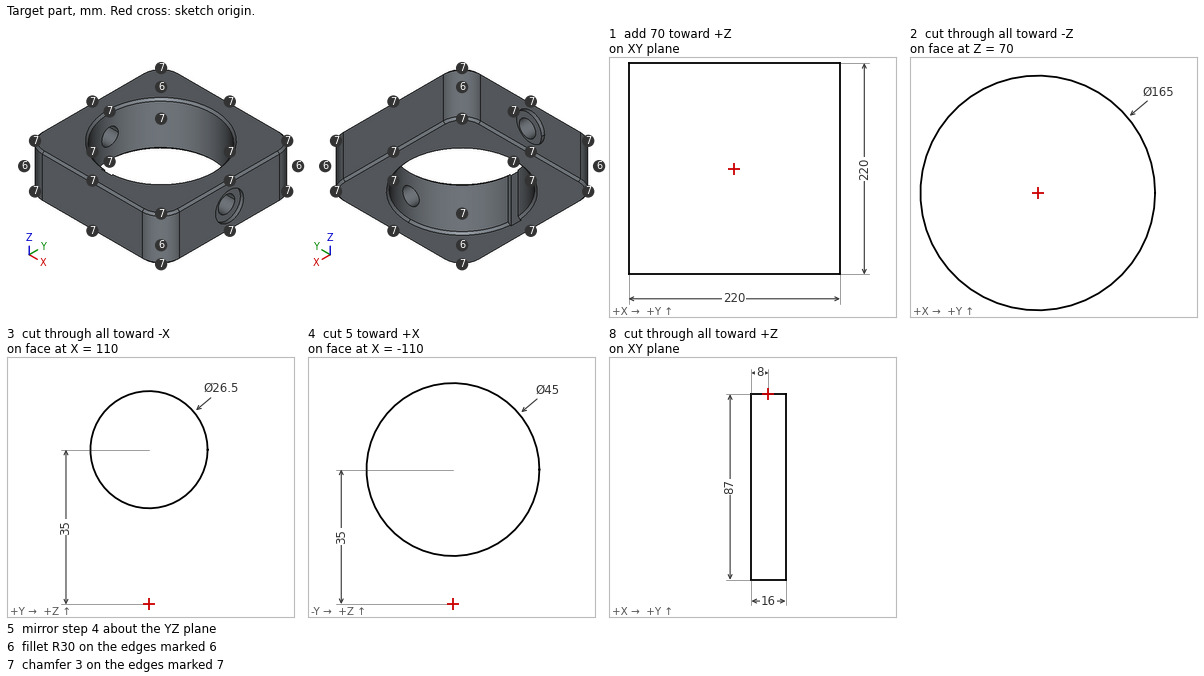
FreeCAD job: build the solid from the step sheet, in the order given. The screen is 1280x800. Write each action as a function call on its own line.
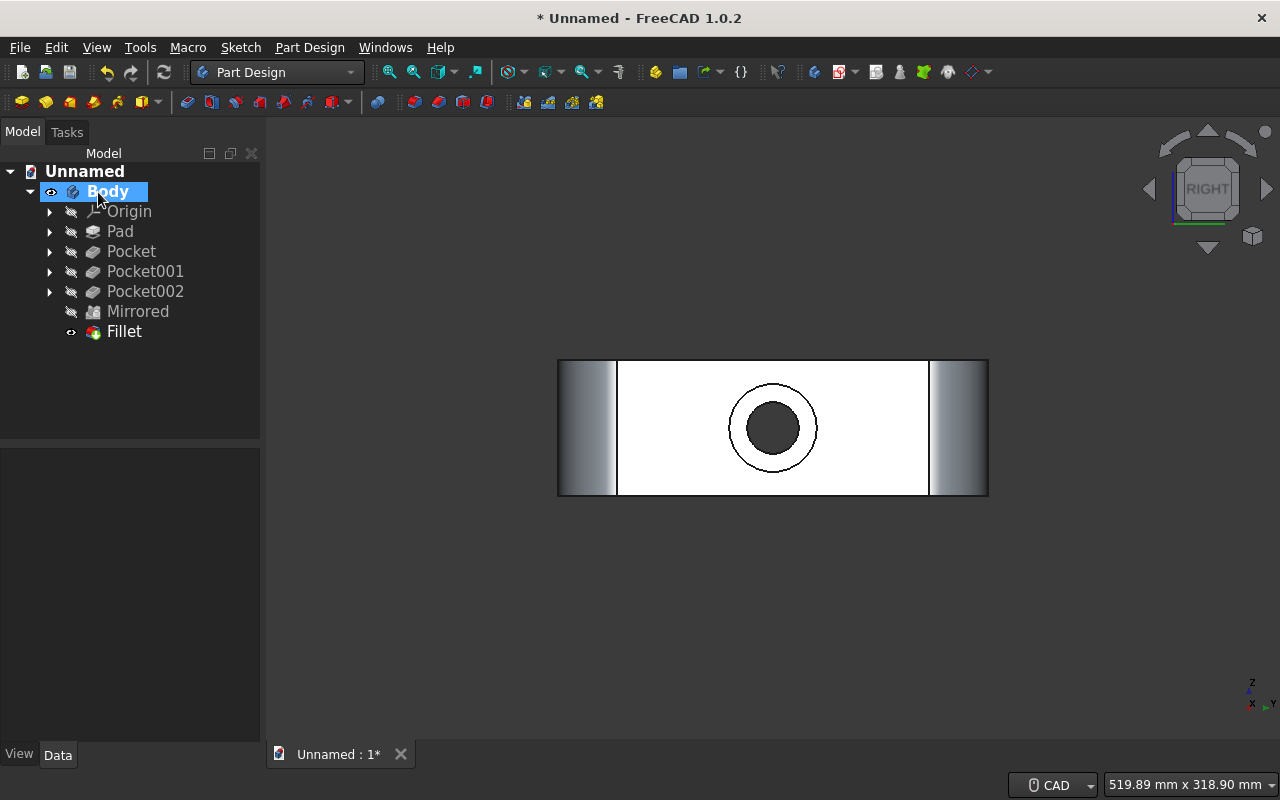
key(v)
key(f)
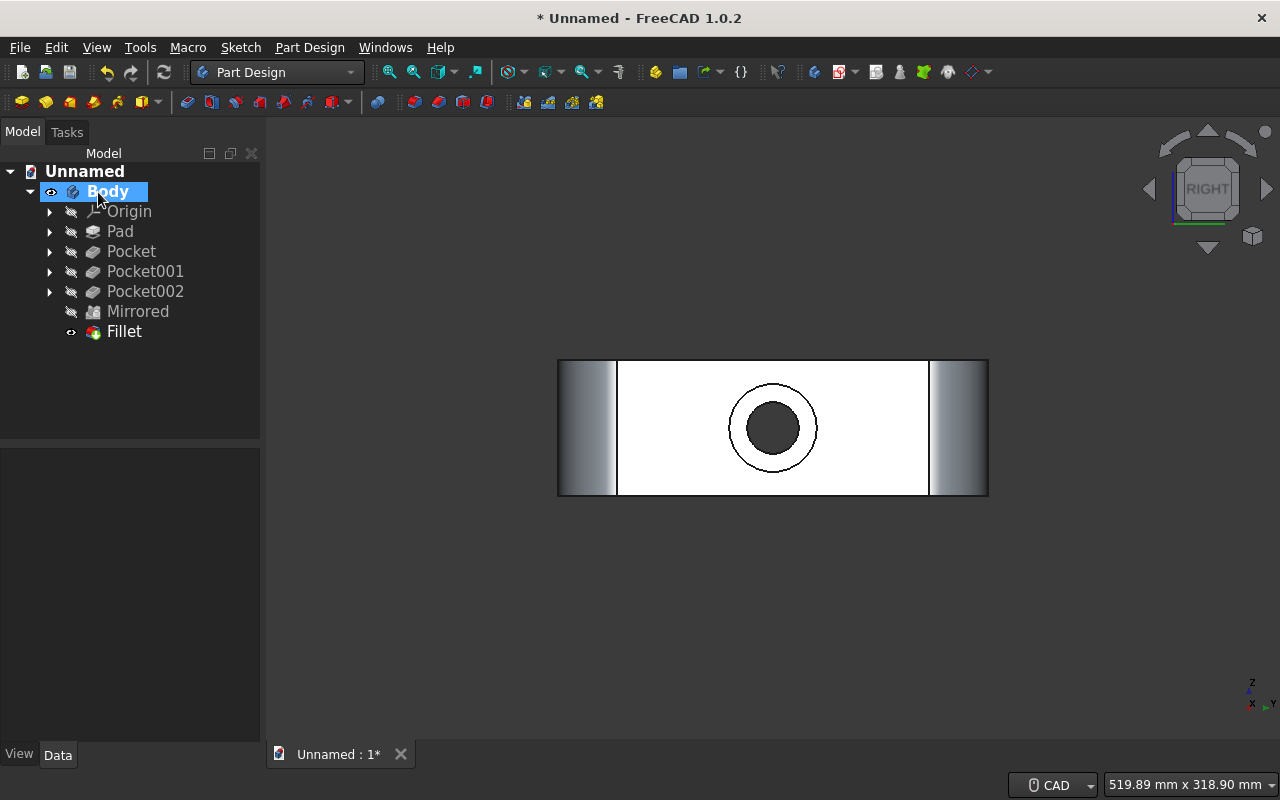
key(0)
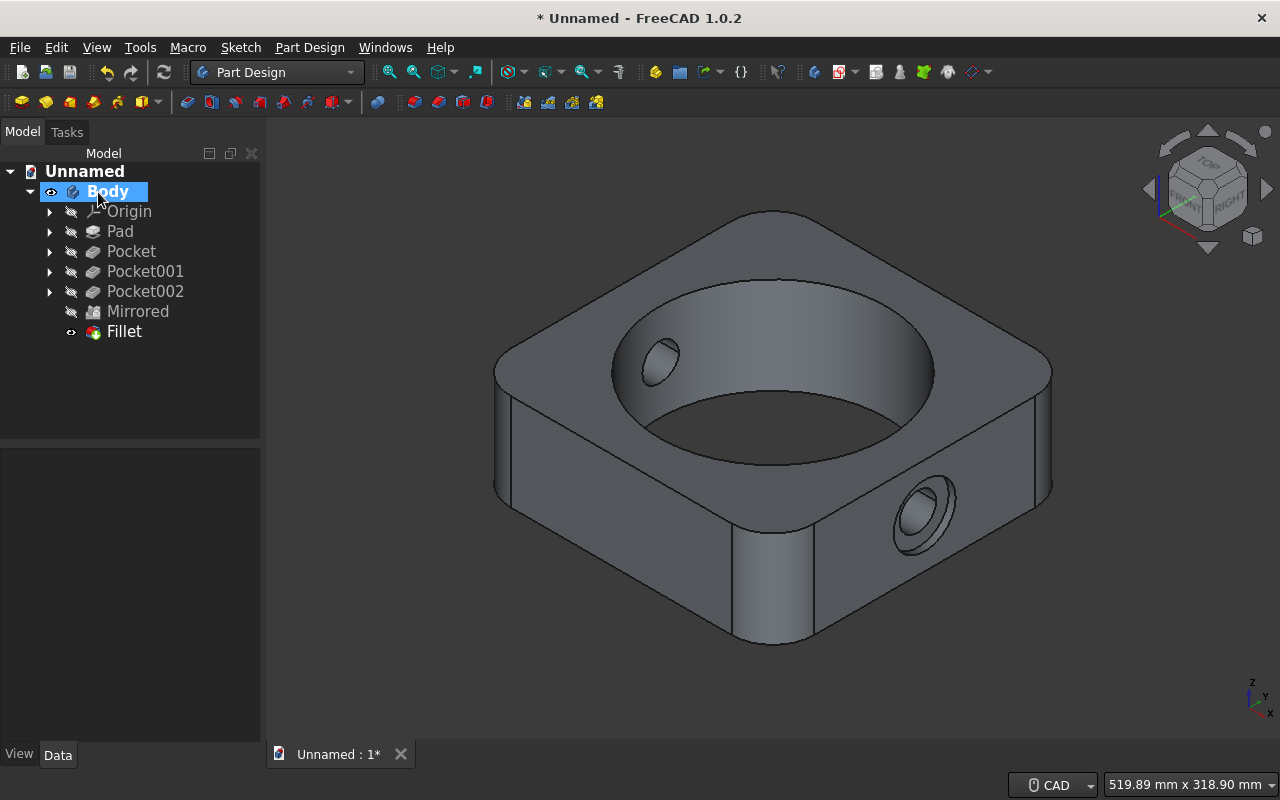
click(990, 396)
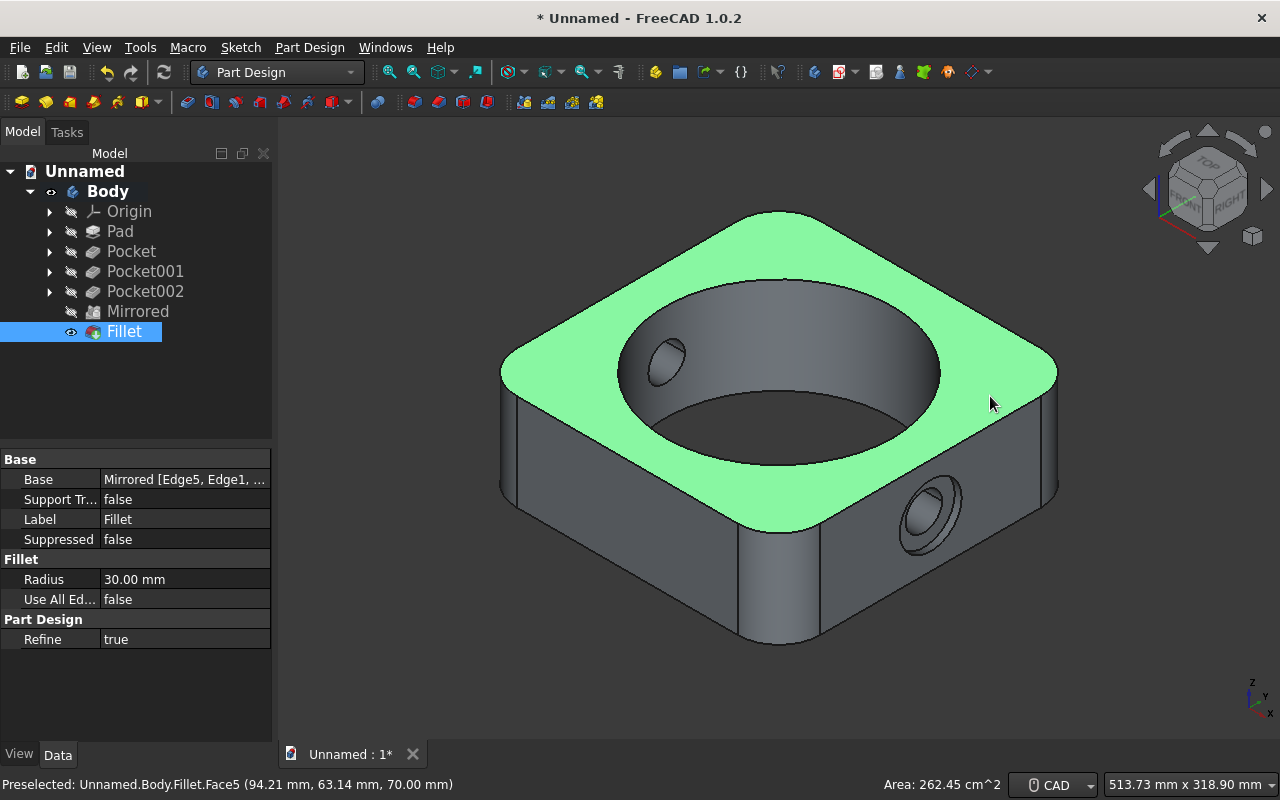
key(2)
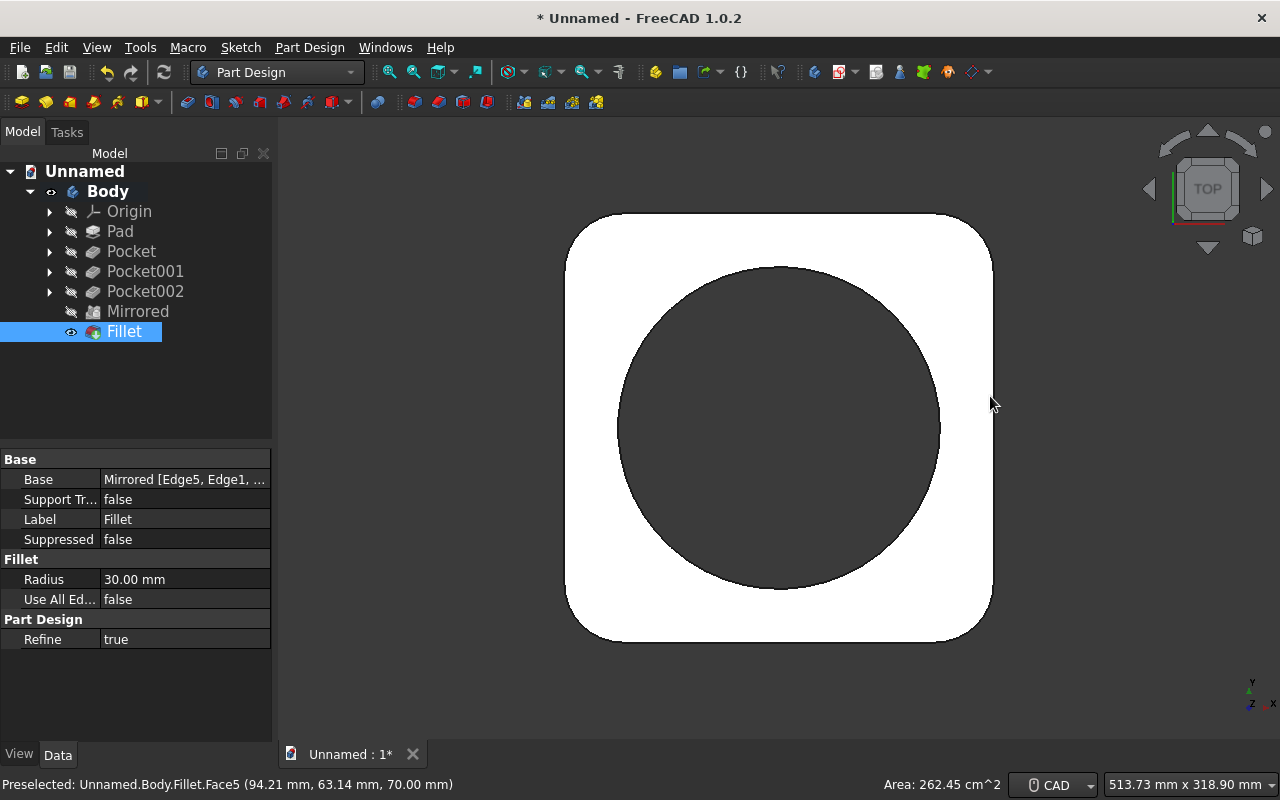
key(1)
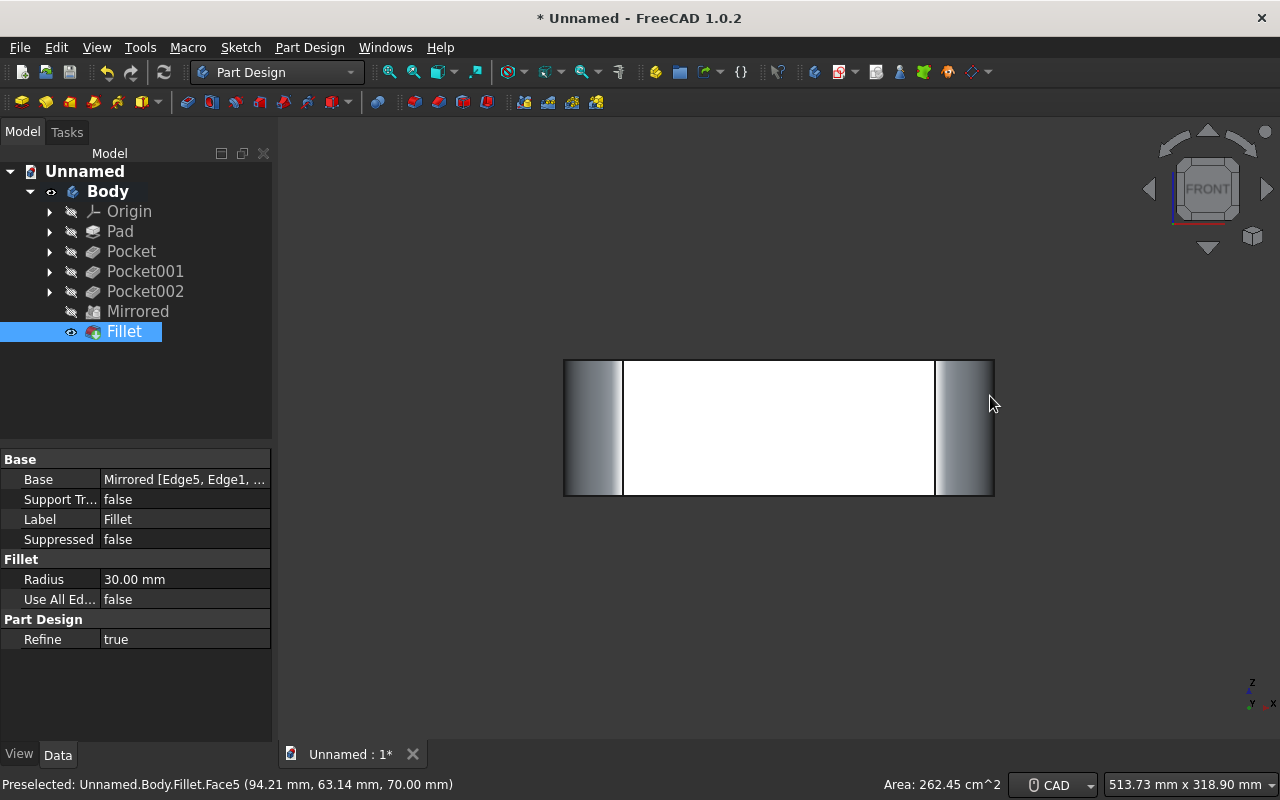
click(390, 72)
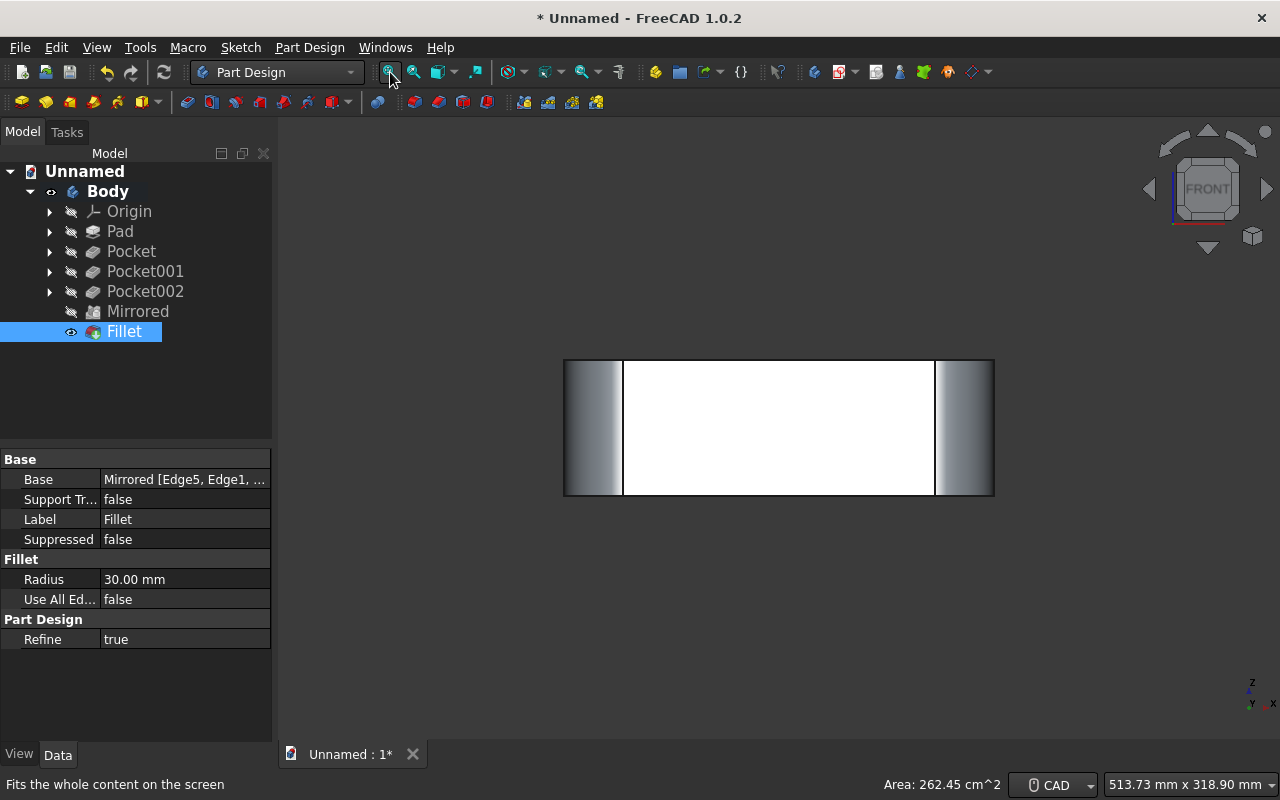
key(3)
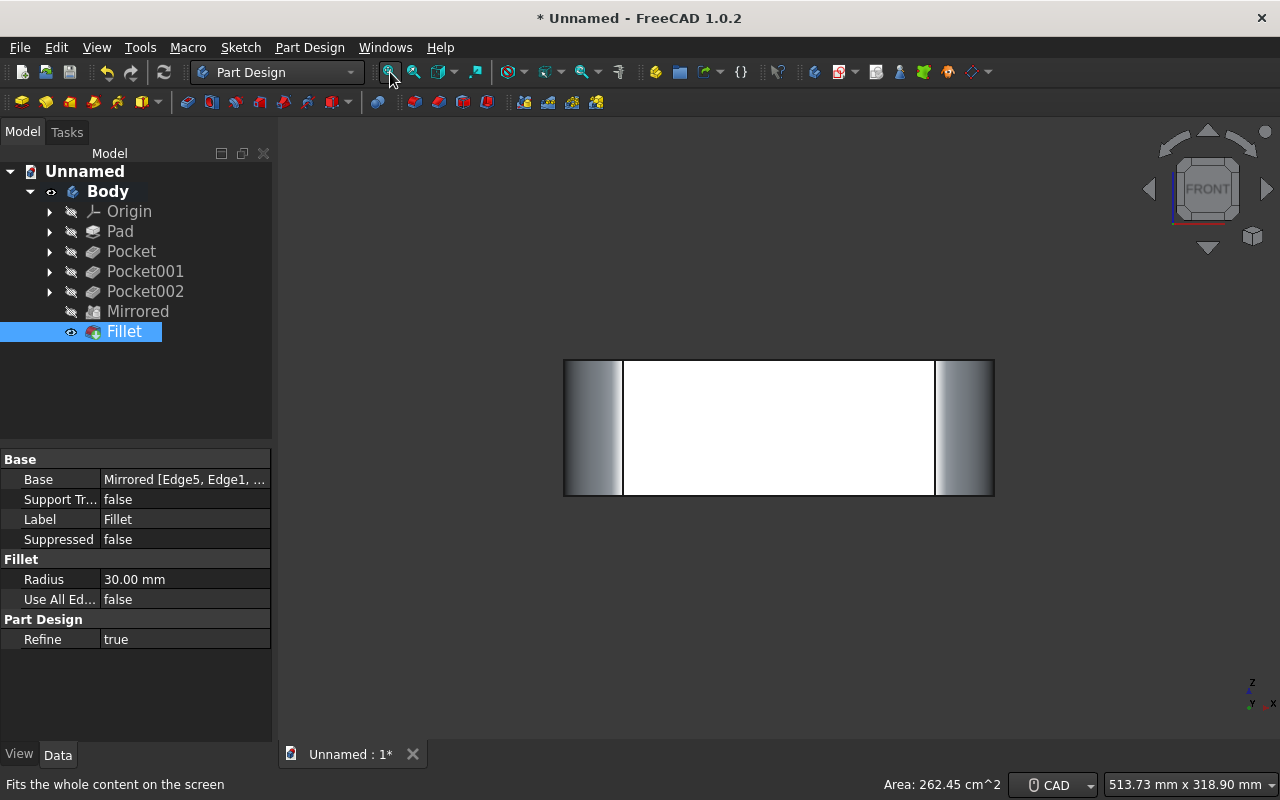
key(v)
key(f)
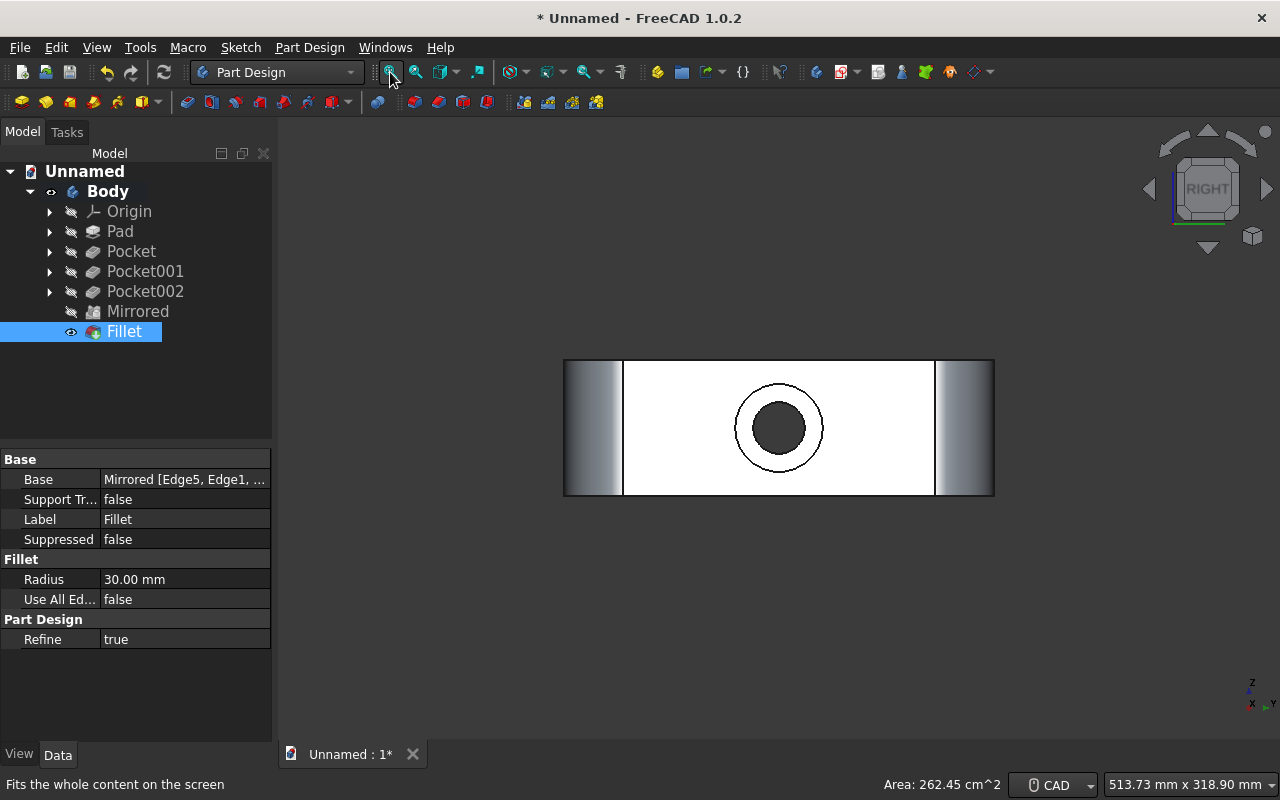
key(5)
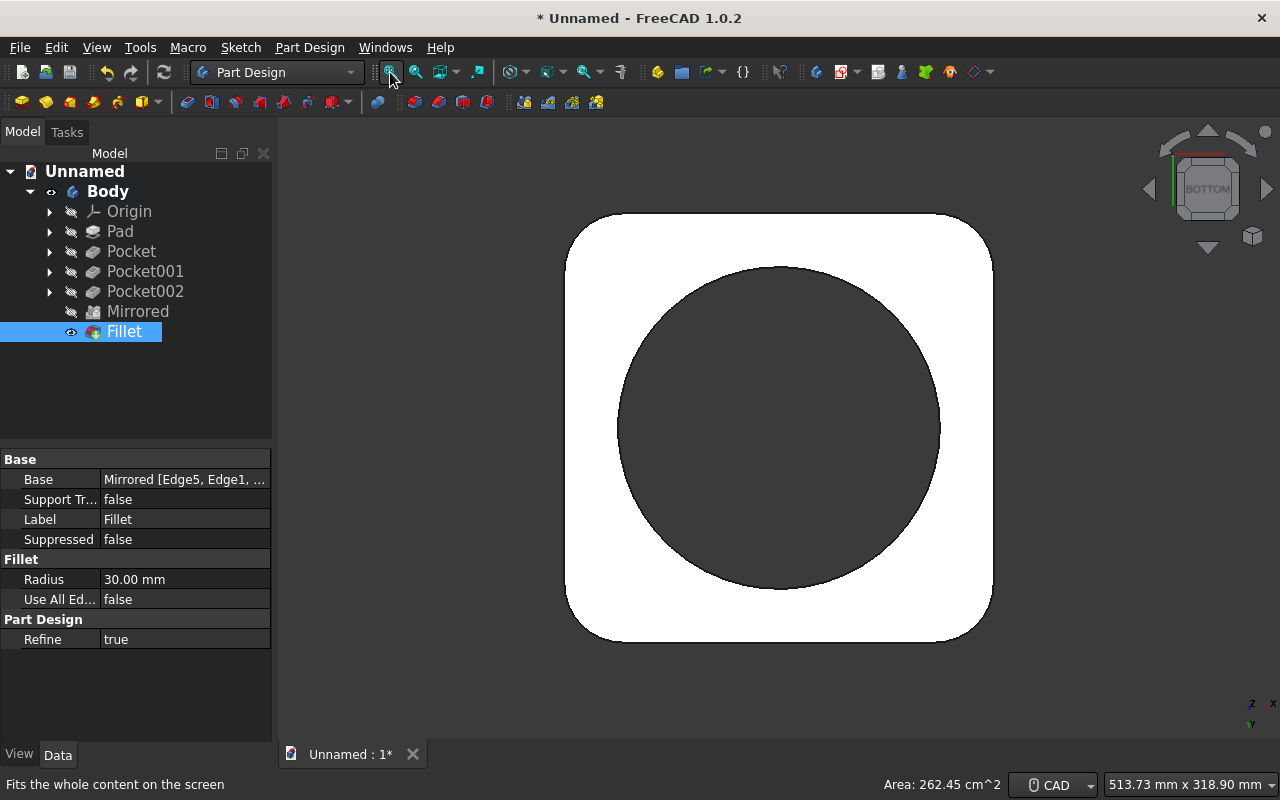
click(963, 550, ctrl)